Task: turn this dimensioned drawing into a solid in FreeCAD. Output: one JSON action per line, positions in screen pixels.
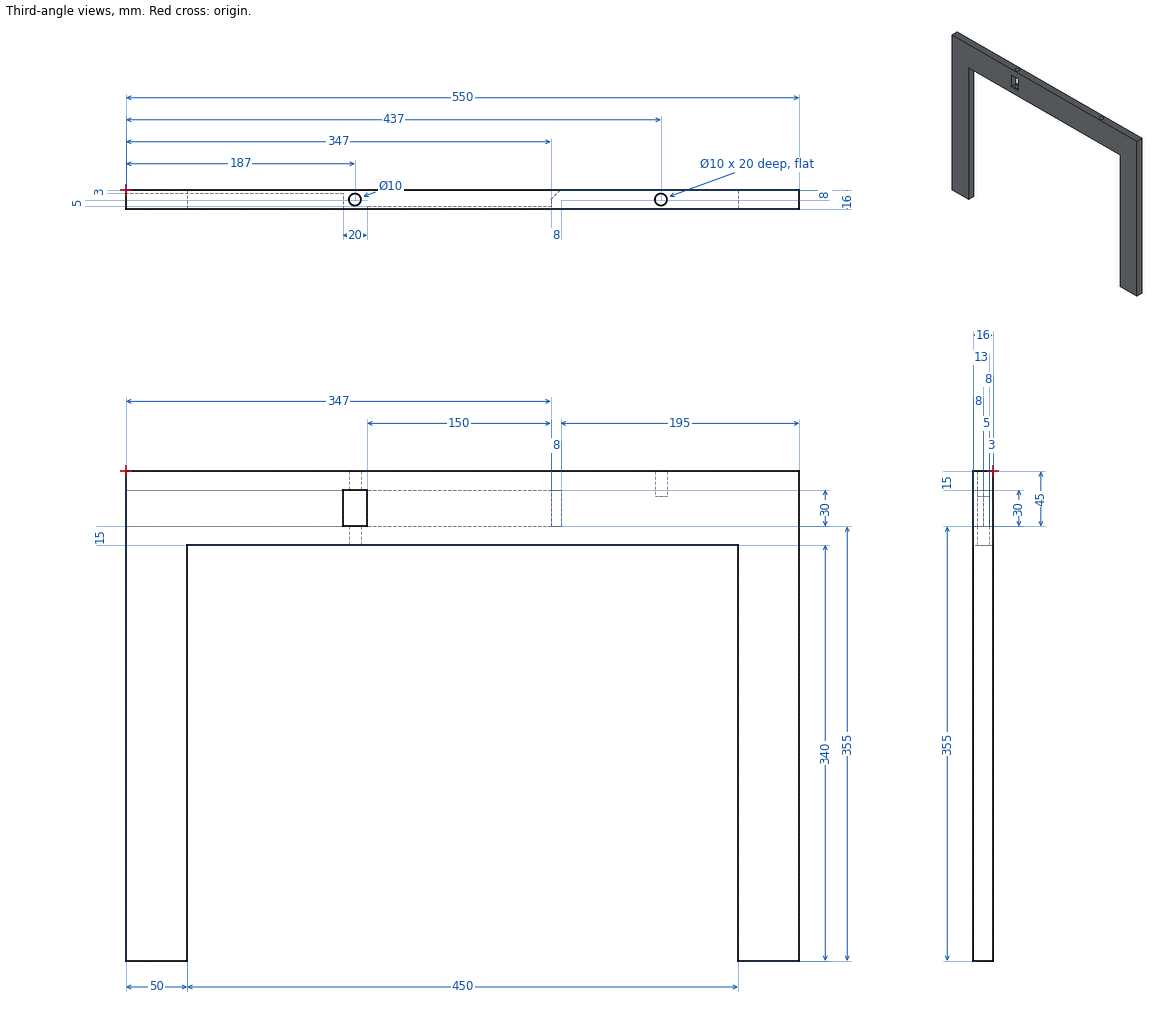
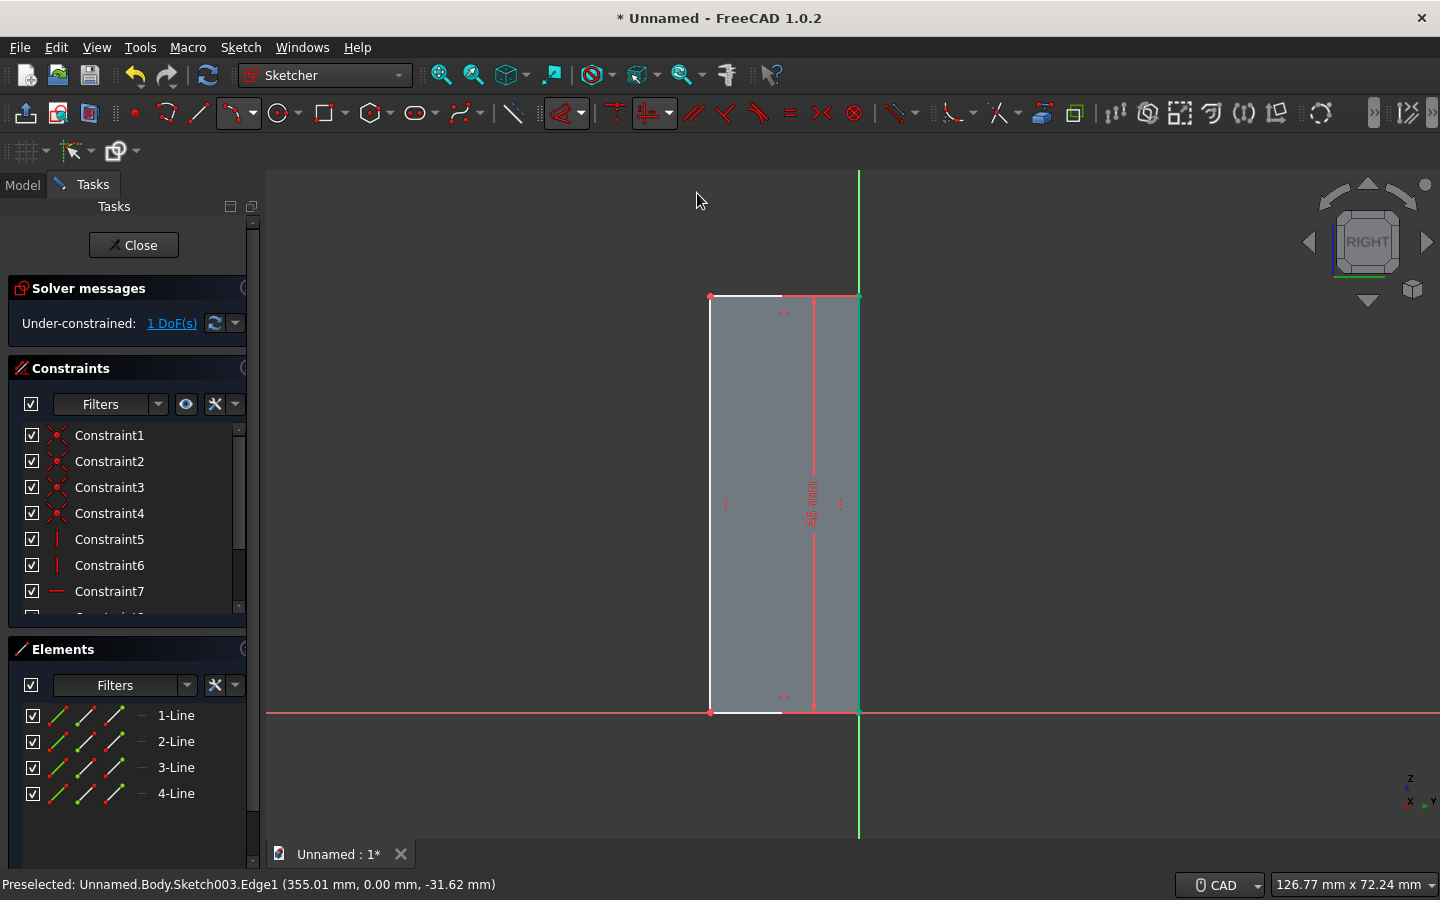
{"action": "left_click", "coordinate": [814, 296]}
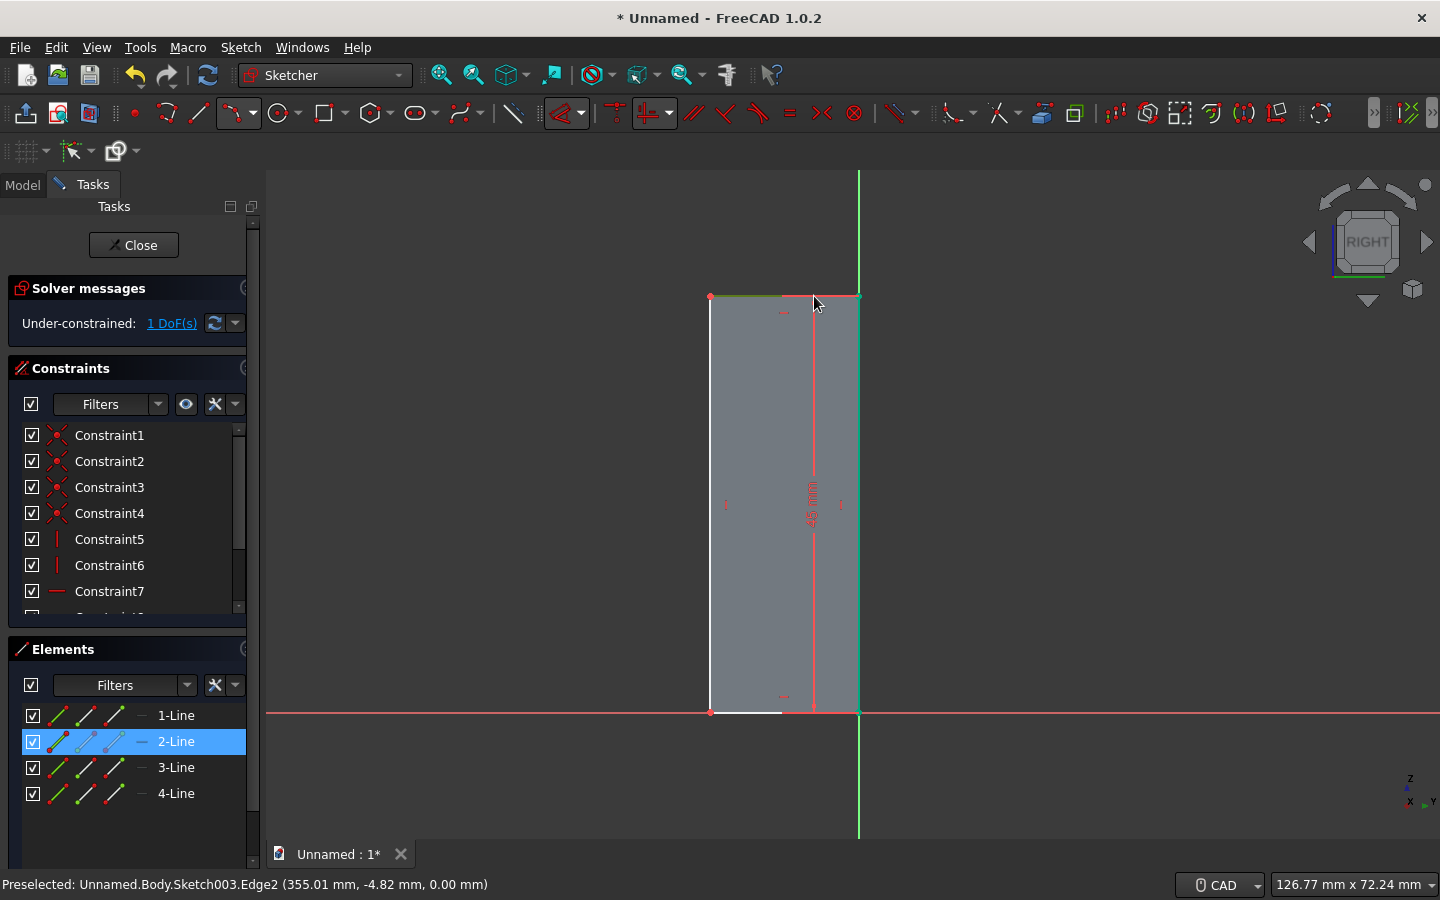
{"action": "key", "text": "l"}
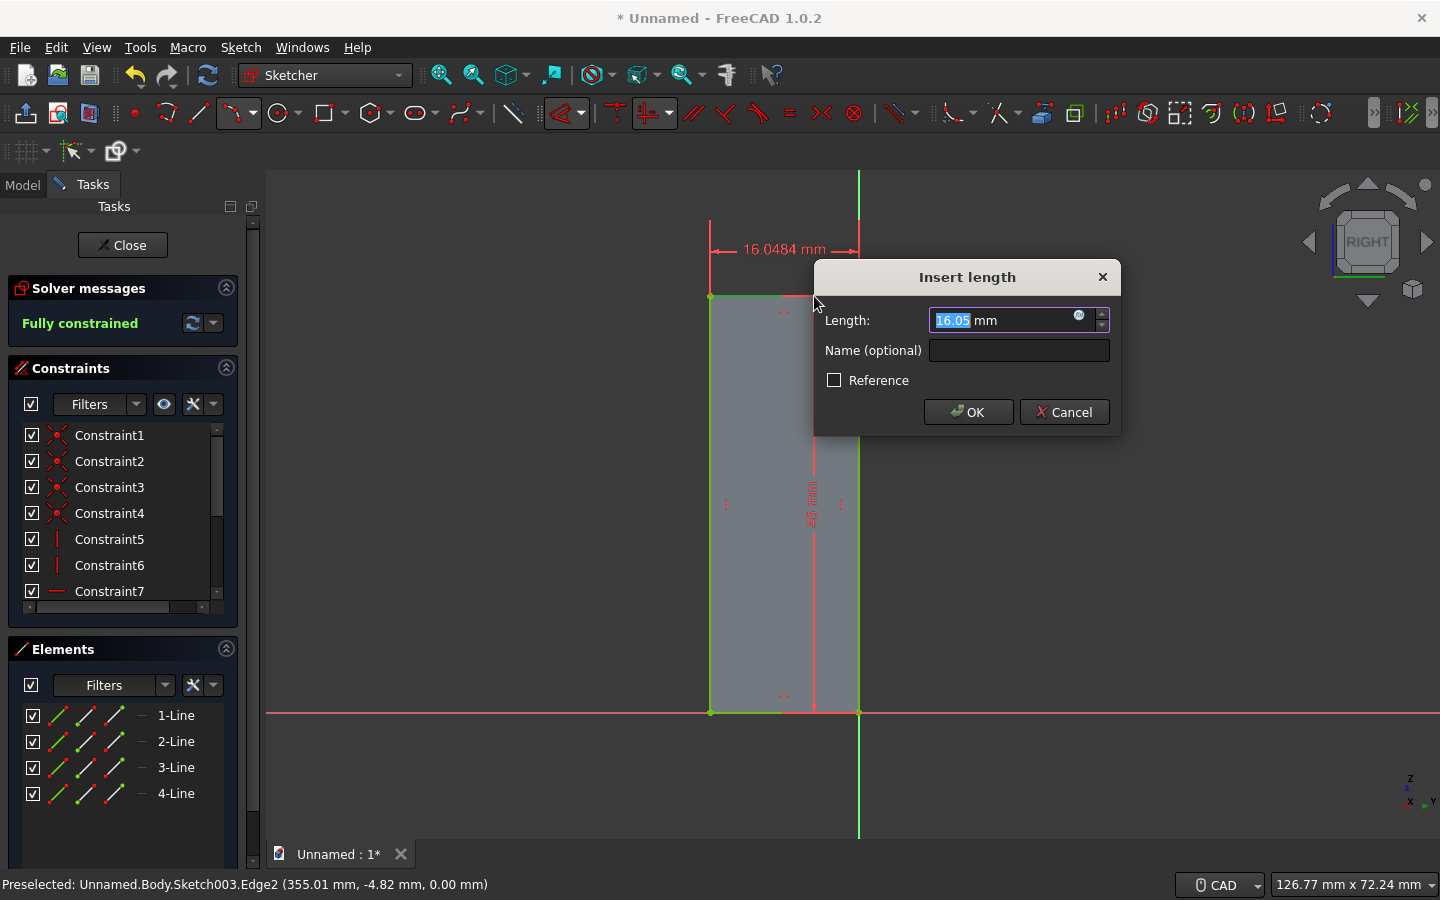
{"action": "type", "text": "16"}
{"action": "key", "text": "Return"}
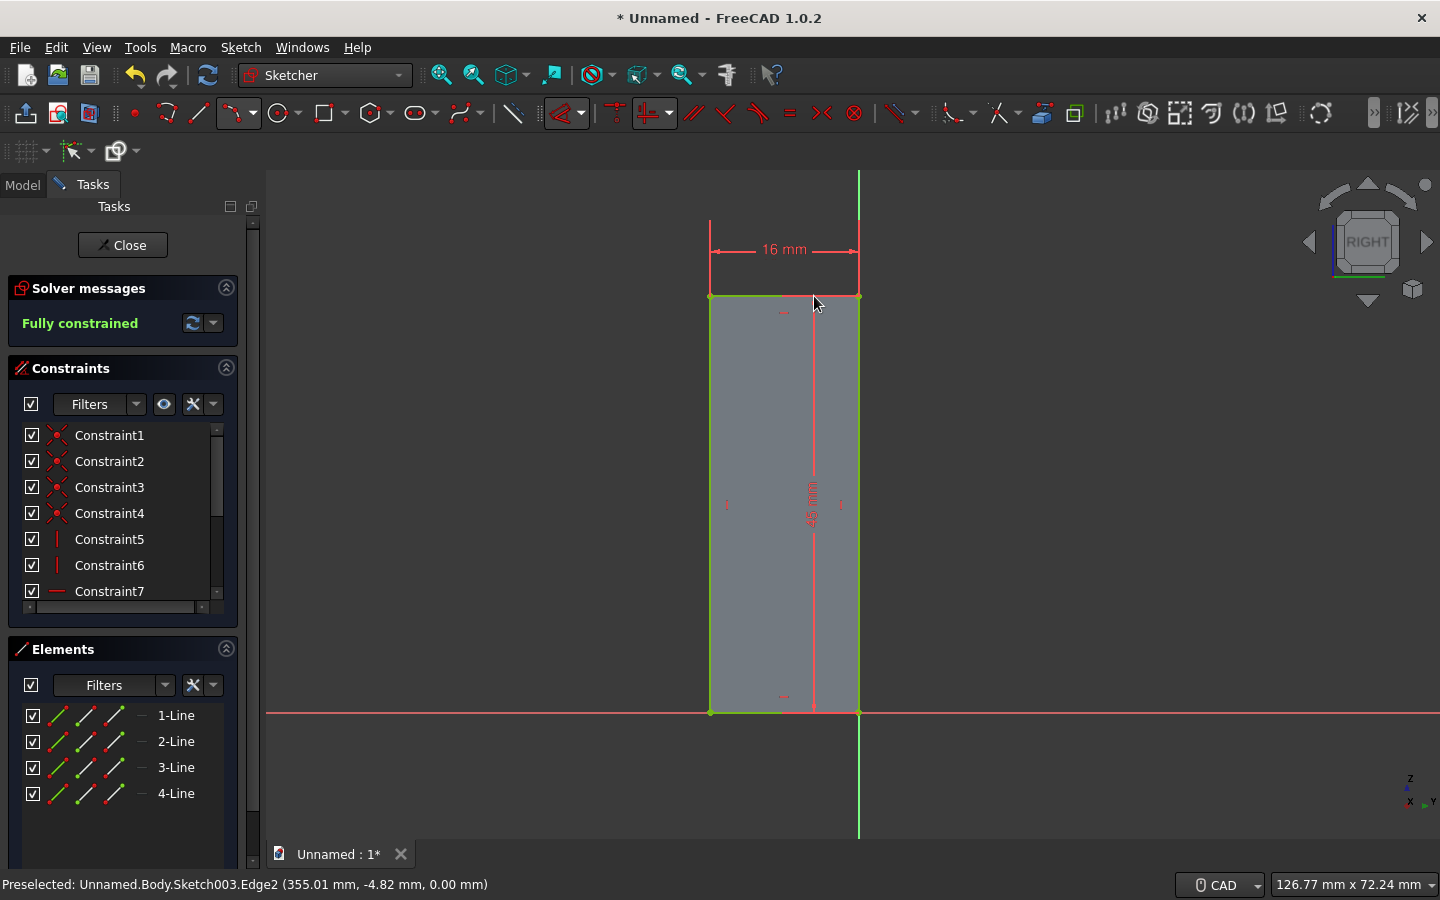
{"action": "left_click", "coordinate": [123, 245]}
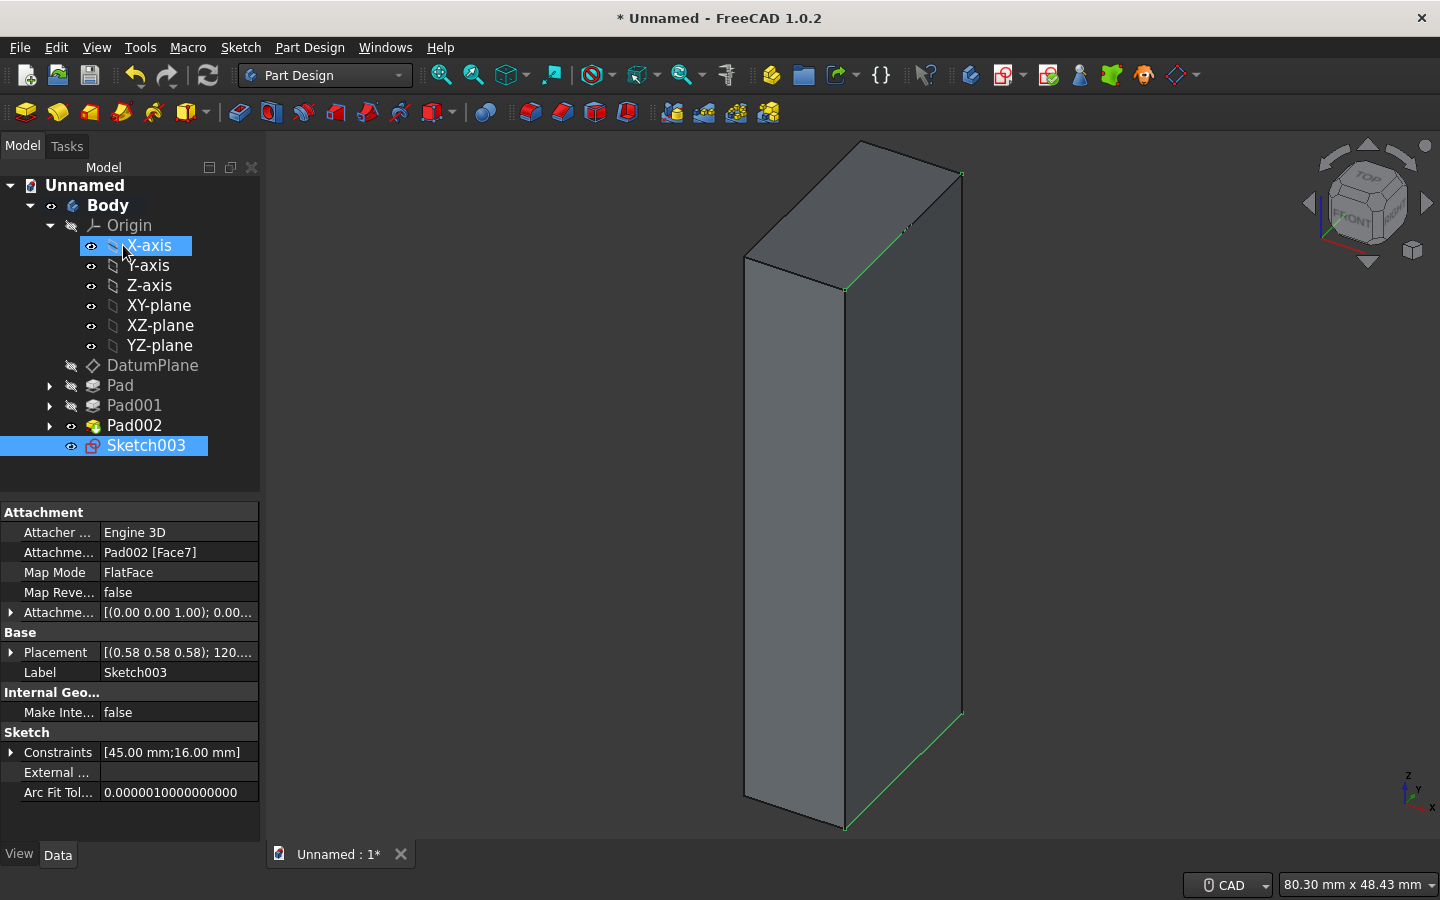
{"action": "left_click", "coordinate": [26, 112]}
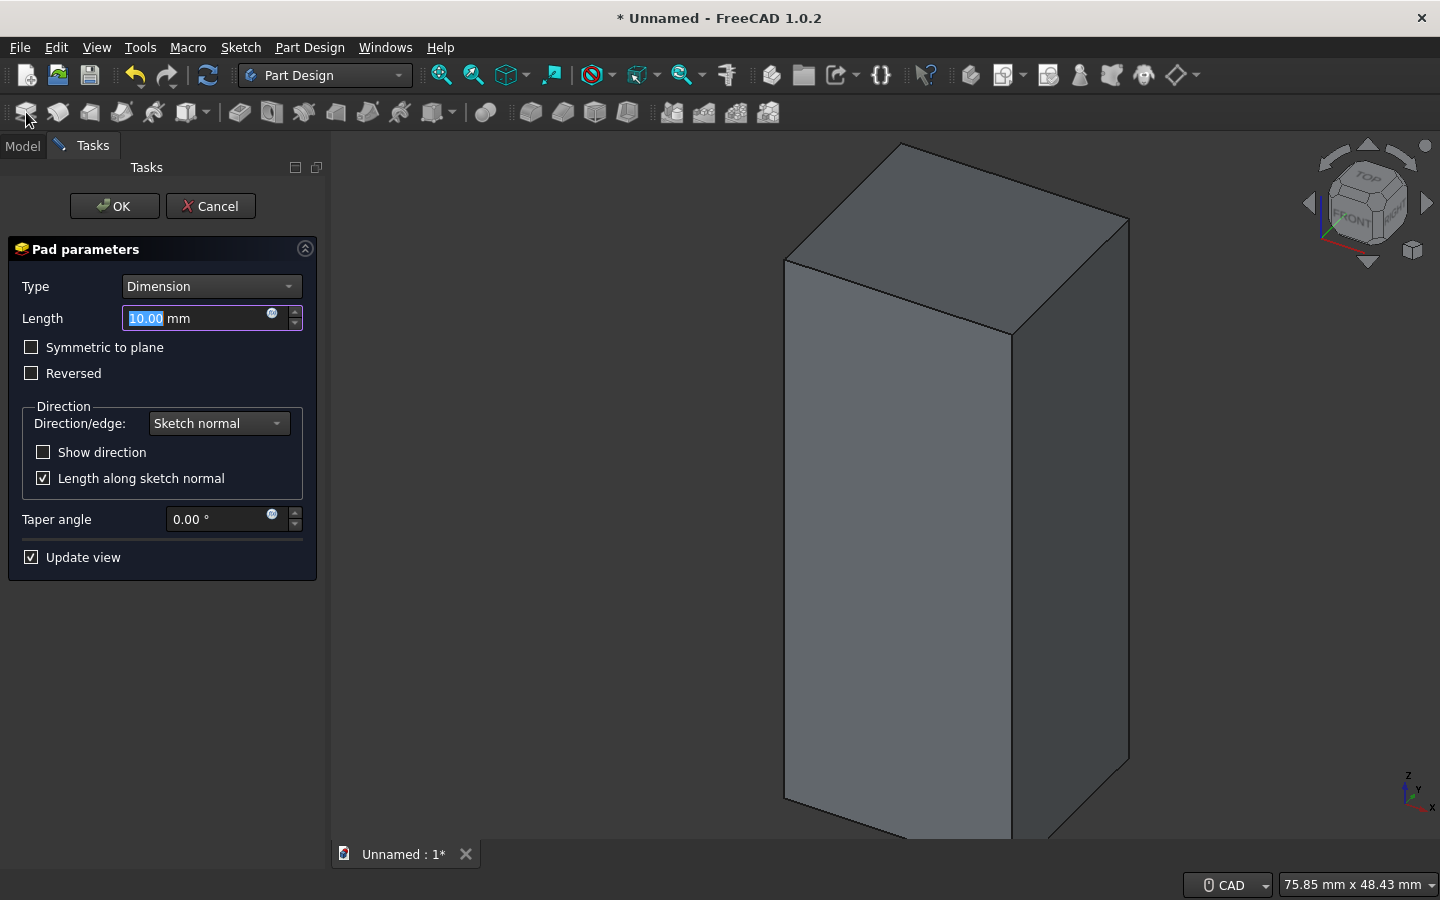
{"action": "type", "text": "195"}
{"action": "key", "text": "Tab"}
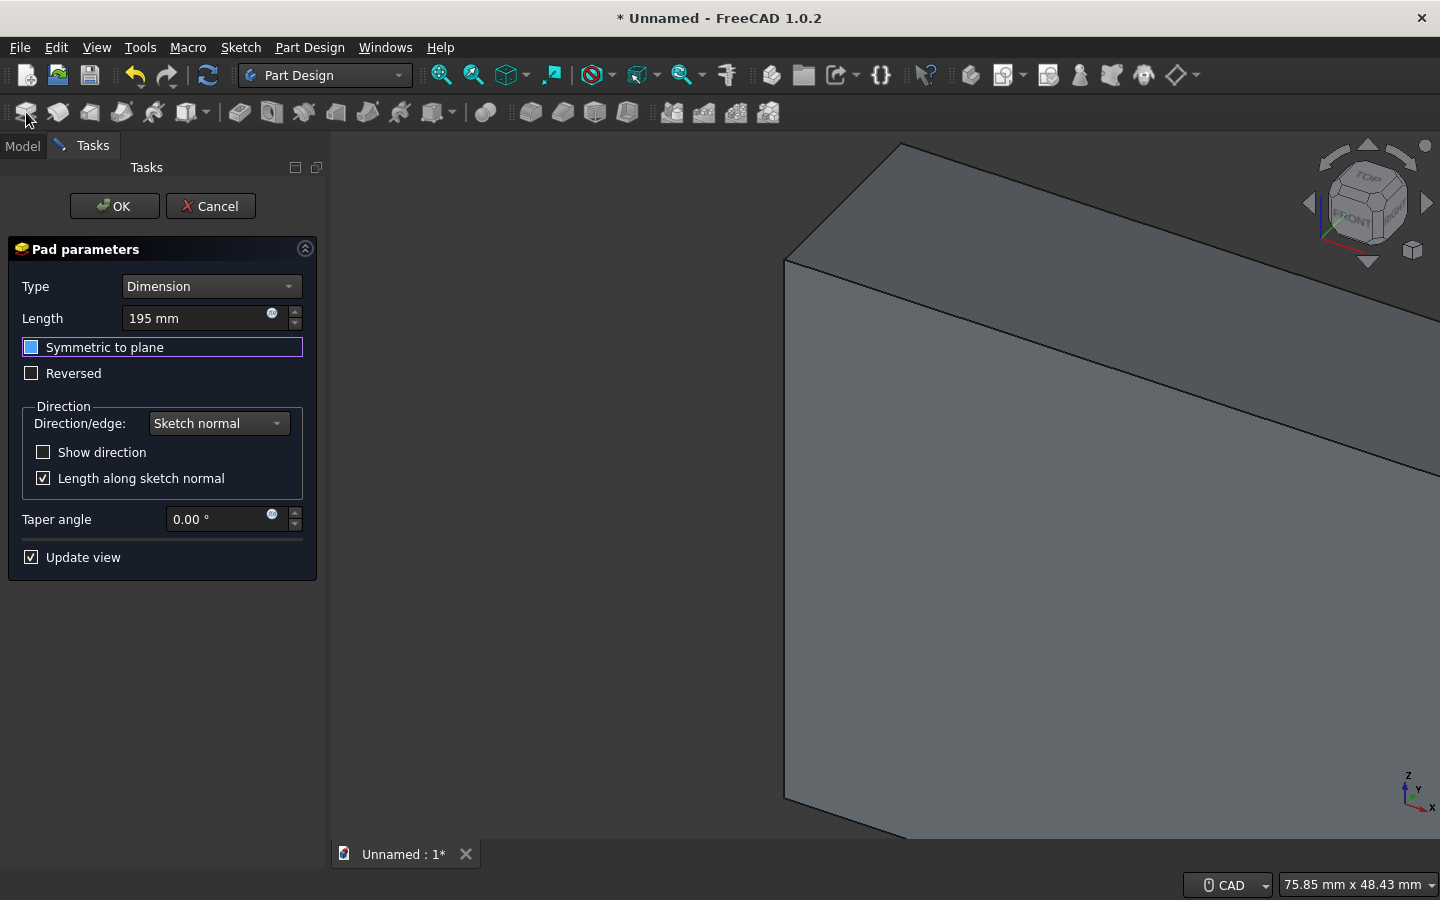
{"action": "left_click", "coordinate": [115, 206]}